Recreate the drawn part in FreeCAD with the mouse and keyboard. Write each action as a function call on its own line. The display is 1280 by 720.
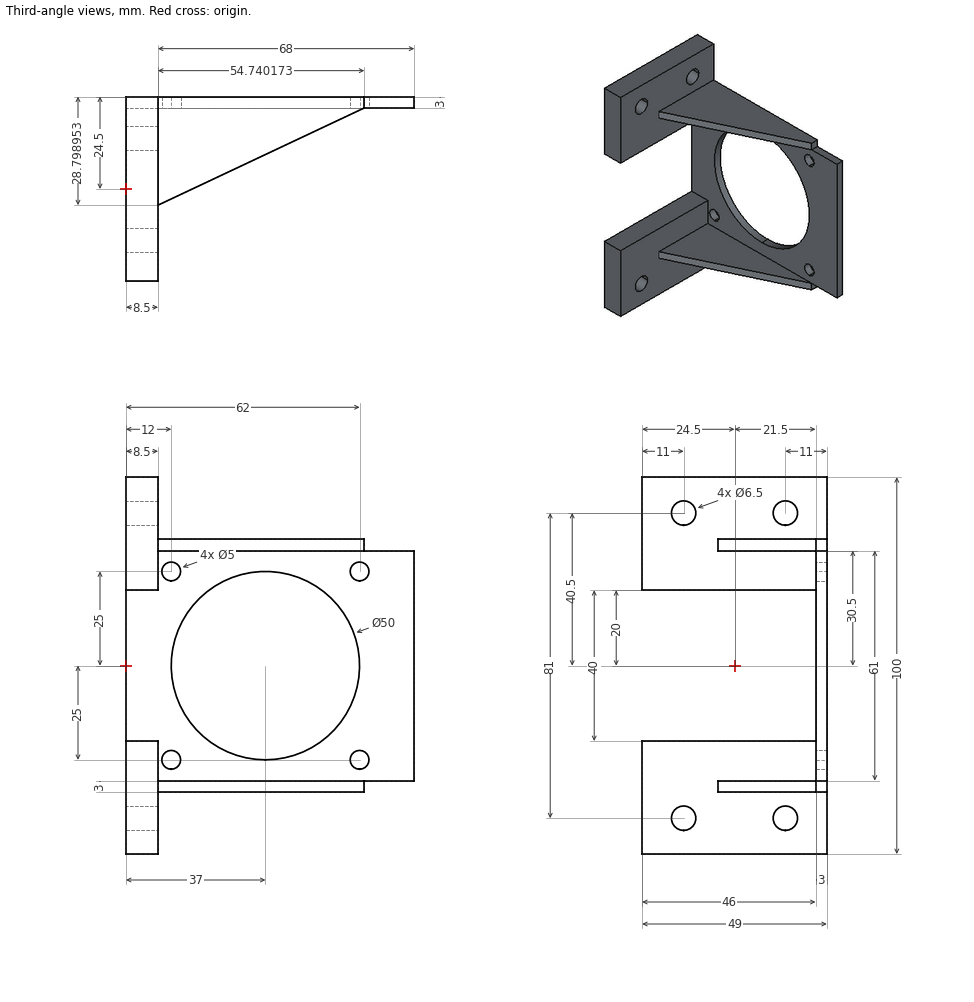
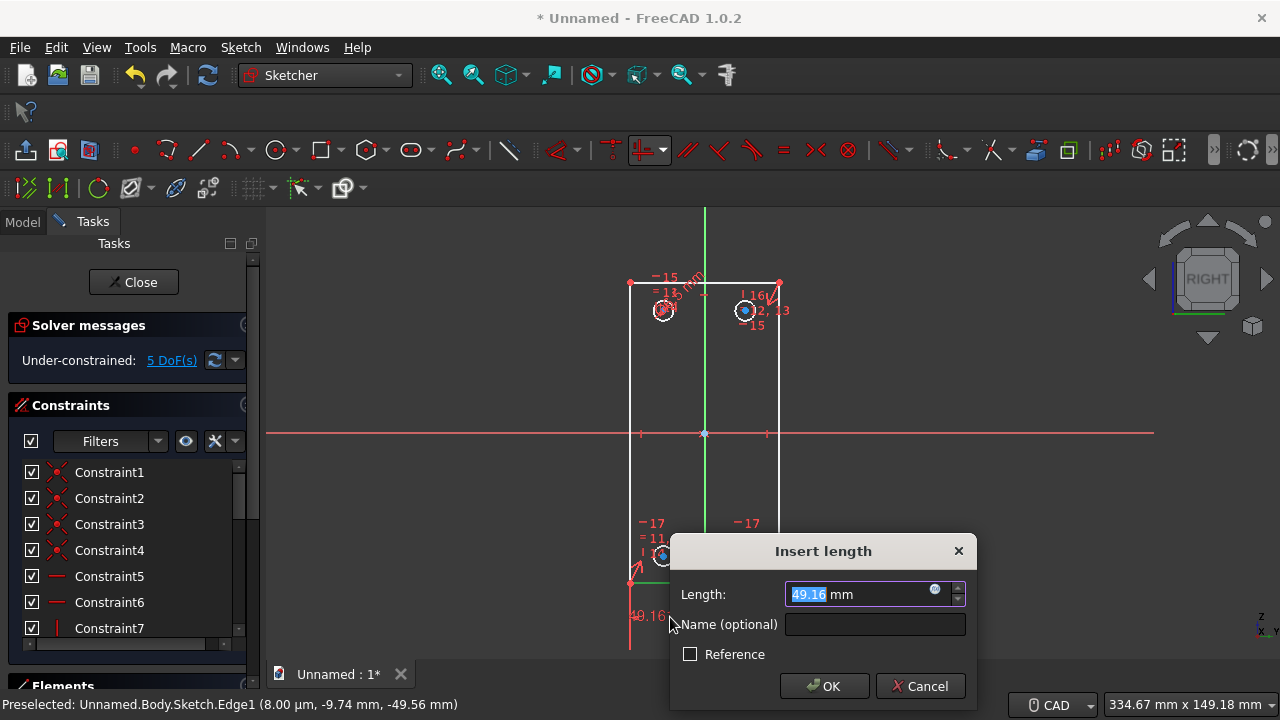
text(49)
key(Return)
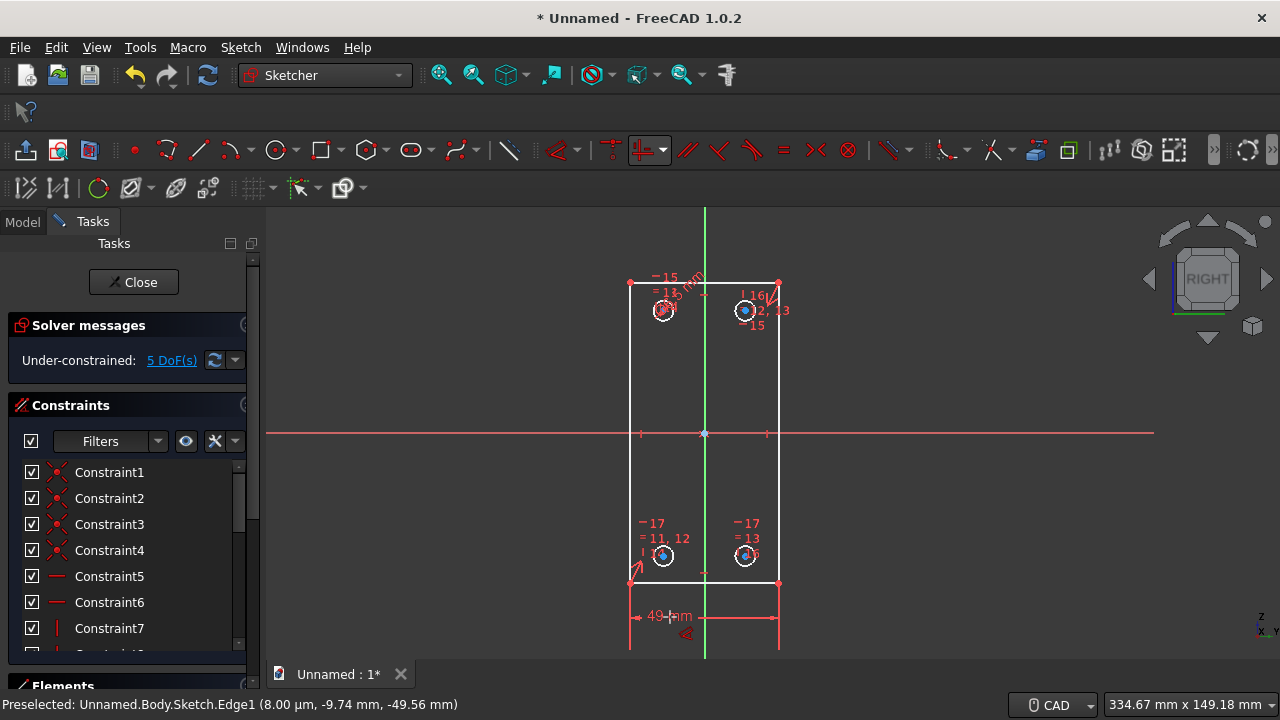
click(779, 493)
click(813, 364)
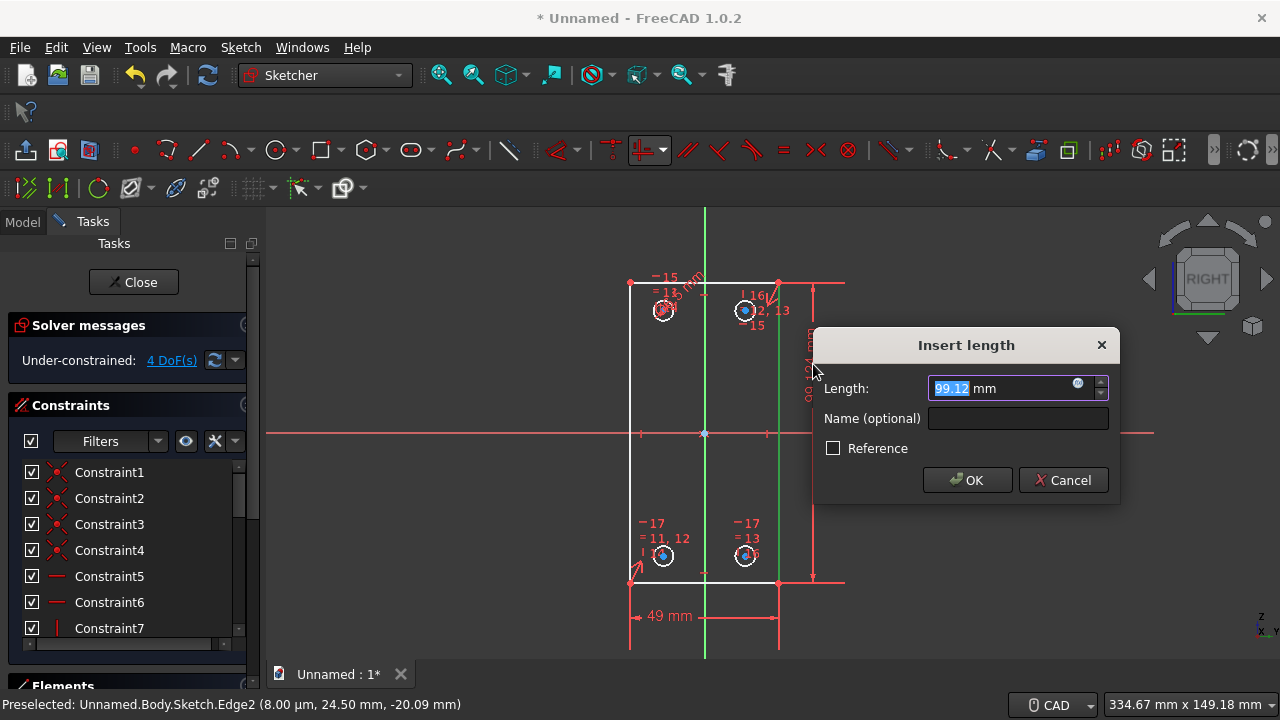
text(100)
key(Return)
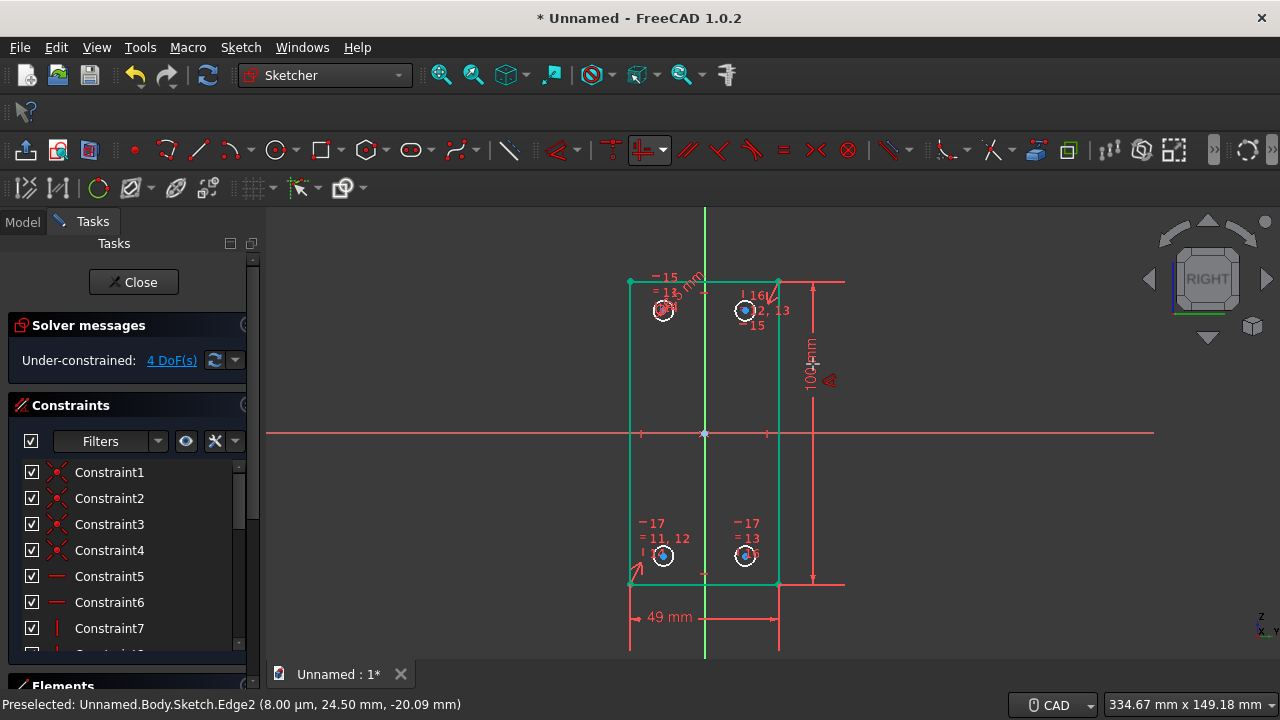
click(630, 282)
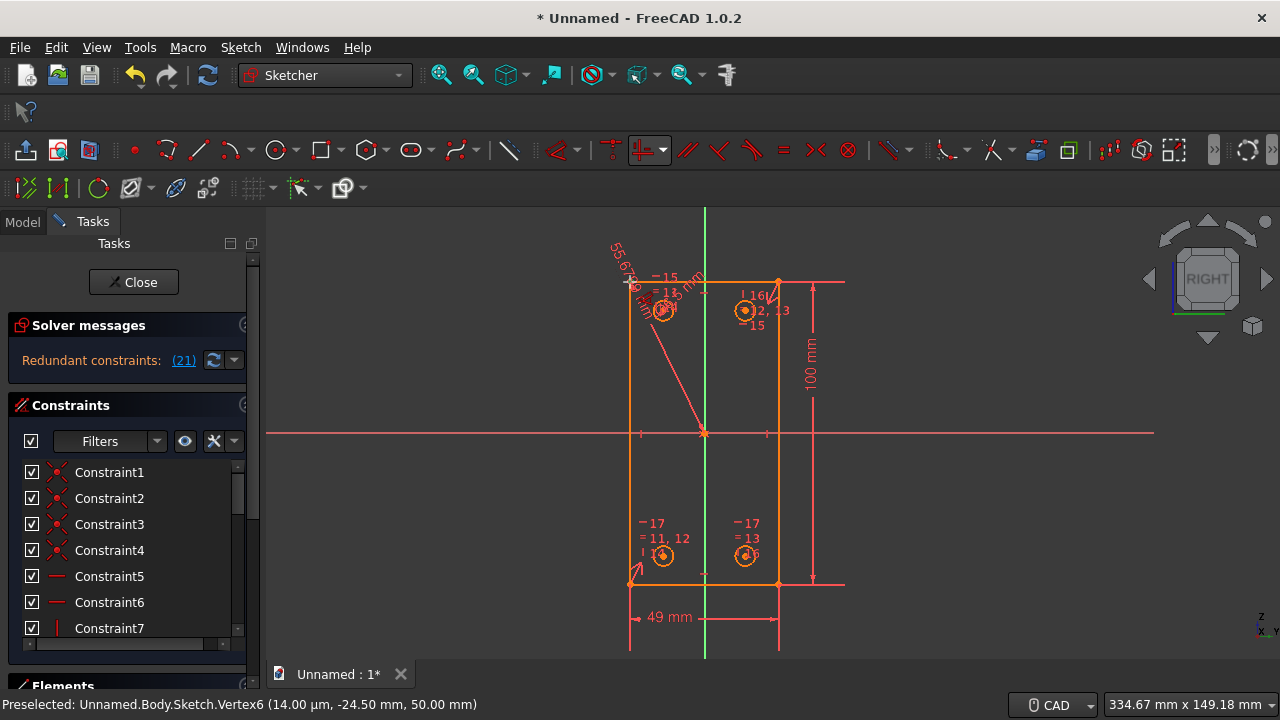
click(664, 311)
click(647, 248)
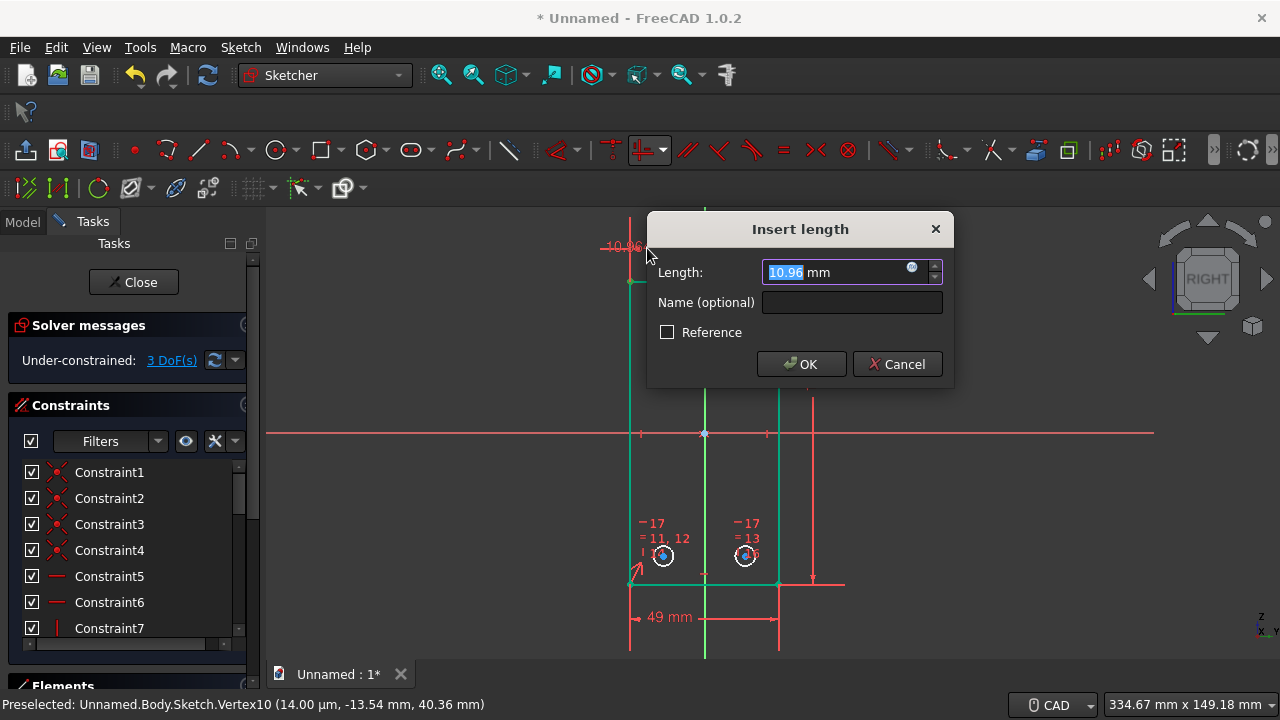
text(11)
key(Return)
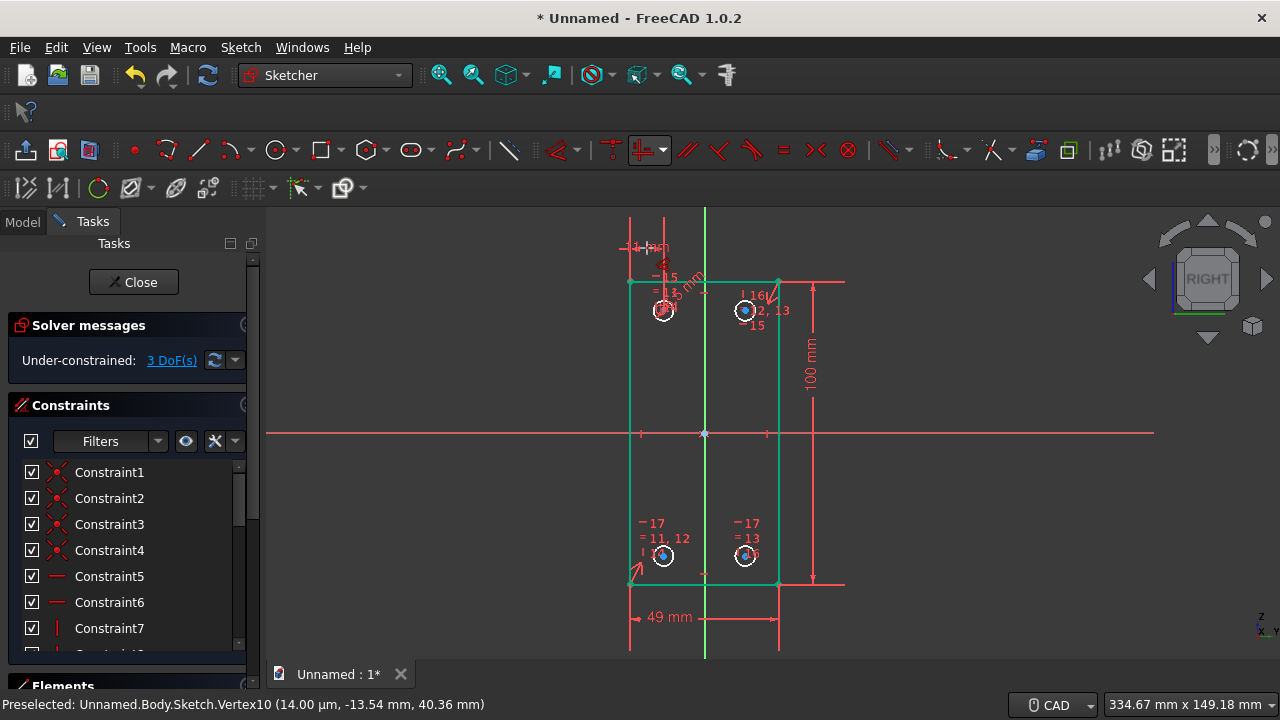
click(664, 311)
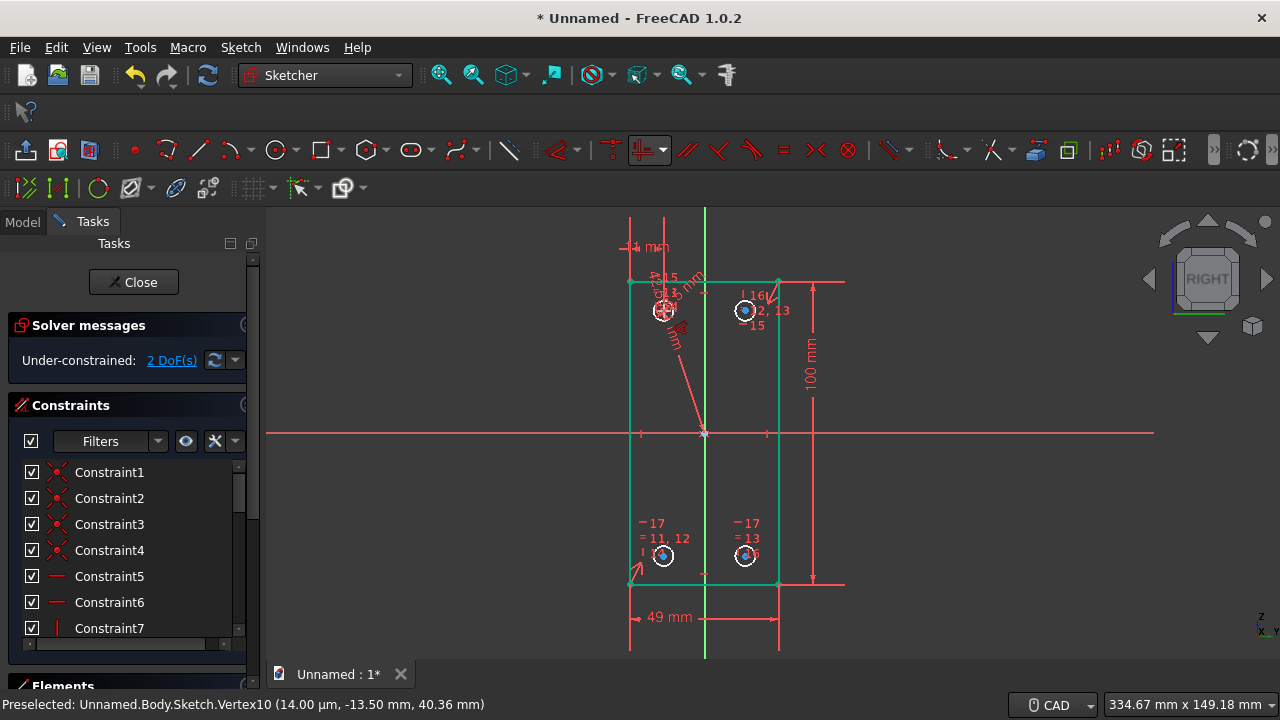
click(664, 556)
click(606, 377)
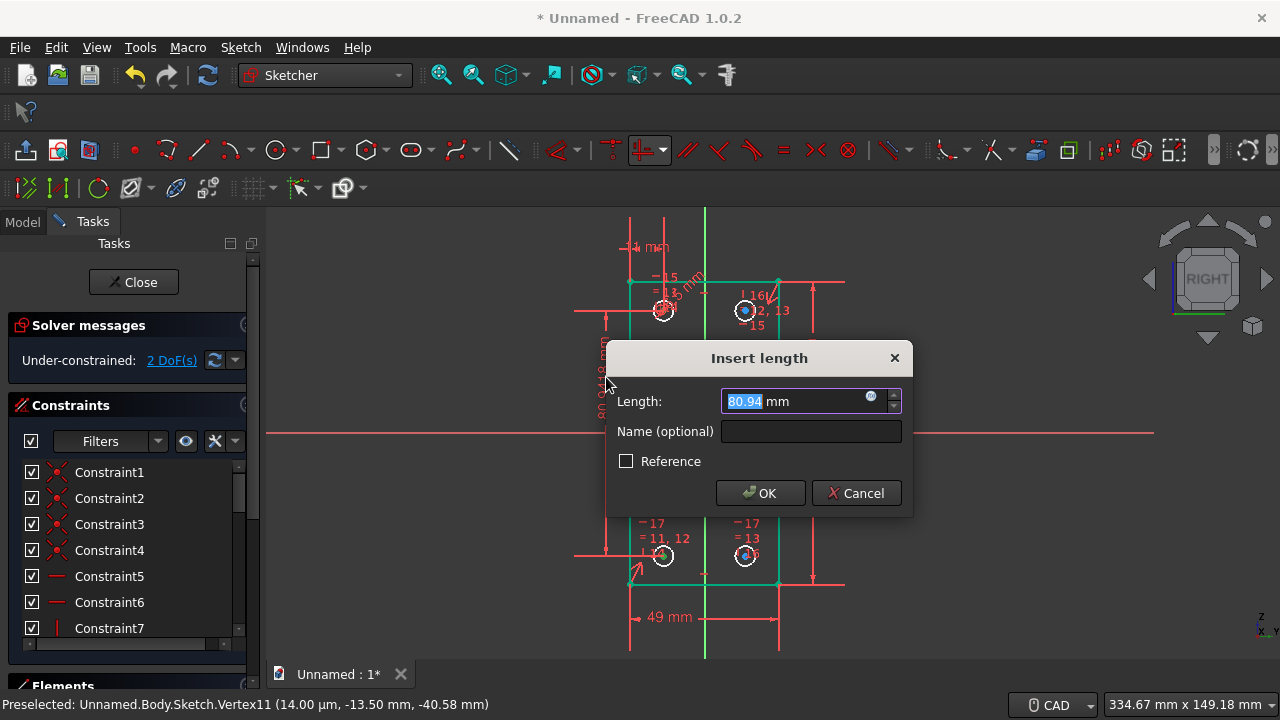
text(81)
key(Return)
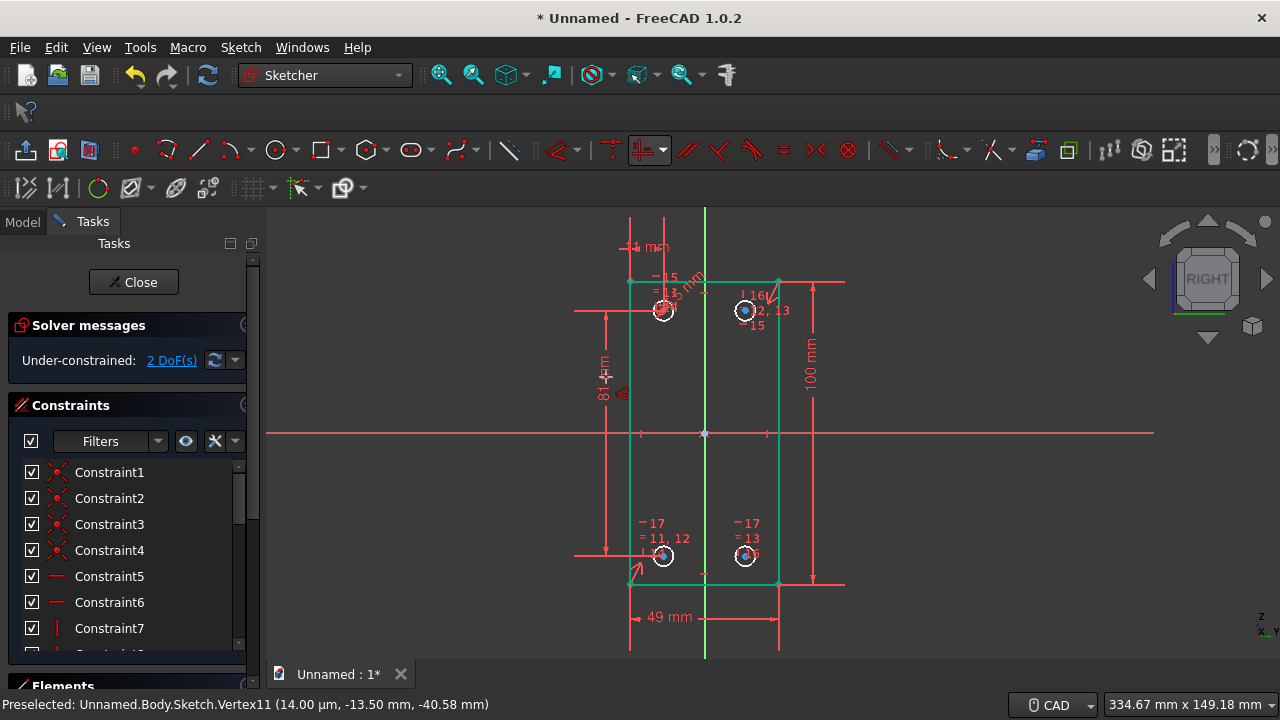
click(779, 282)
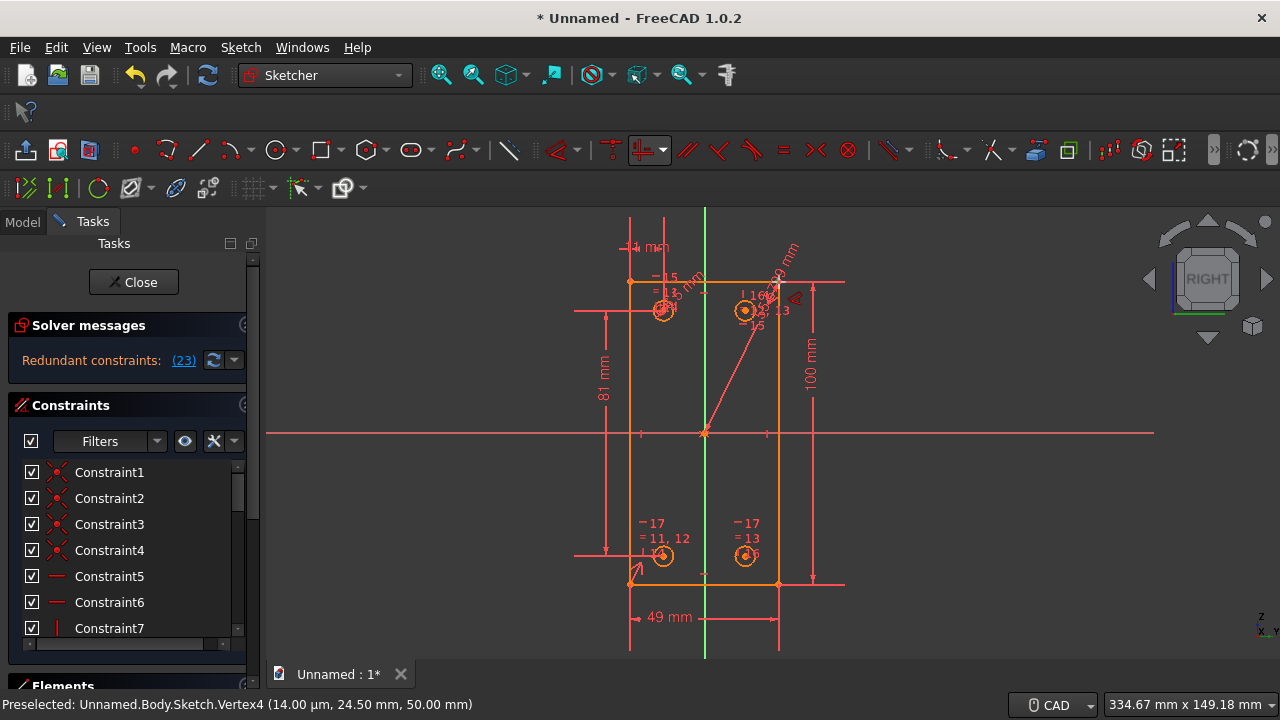
click(745, 311)
click(762, 248)